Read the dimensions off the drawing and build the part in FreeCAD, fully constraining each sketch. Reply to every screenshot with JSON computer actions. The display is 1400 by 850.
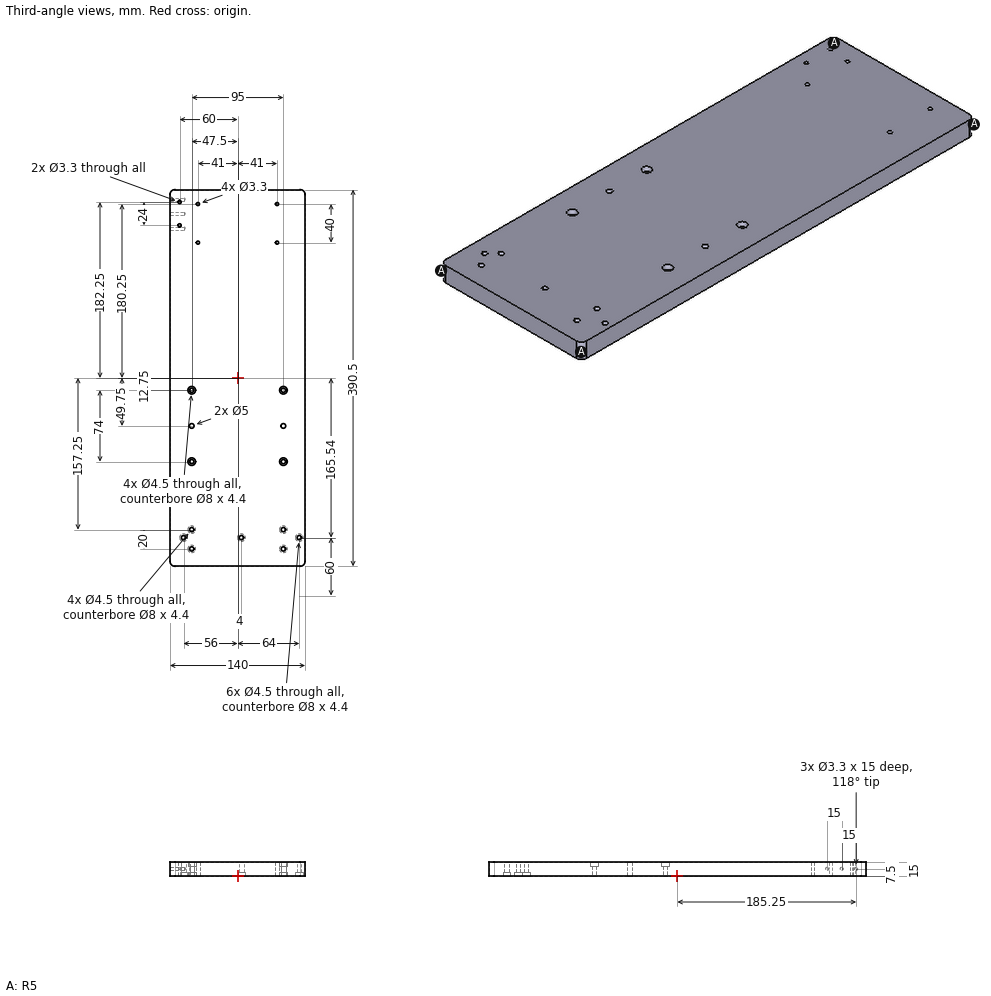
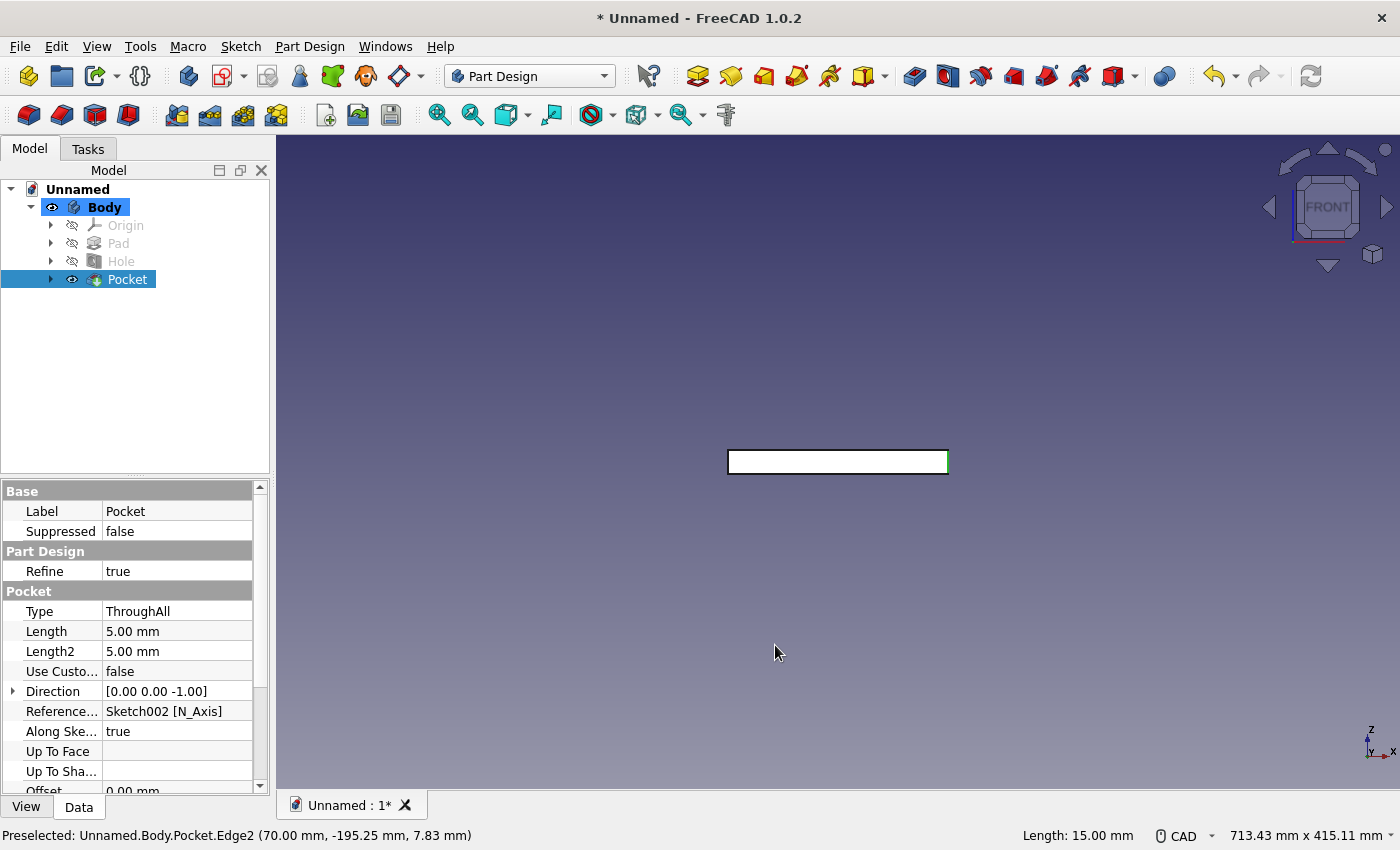
{"action": "key", "text": "v f"}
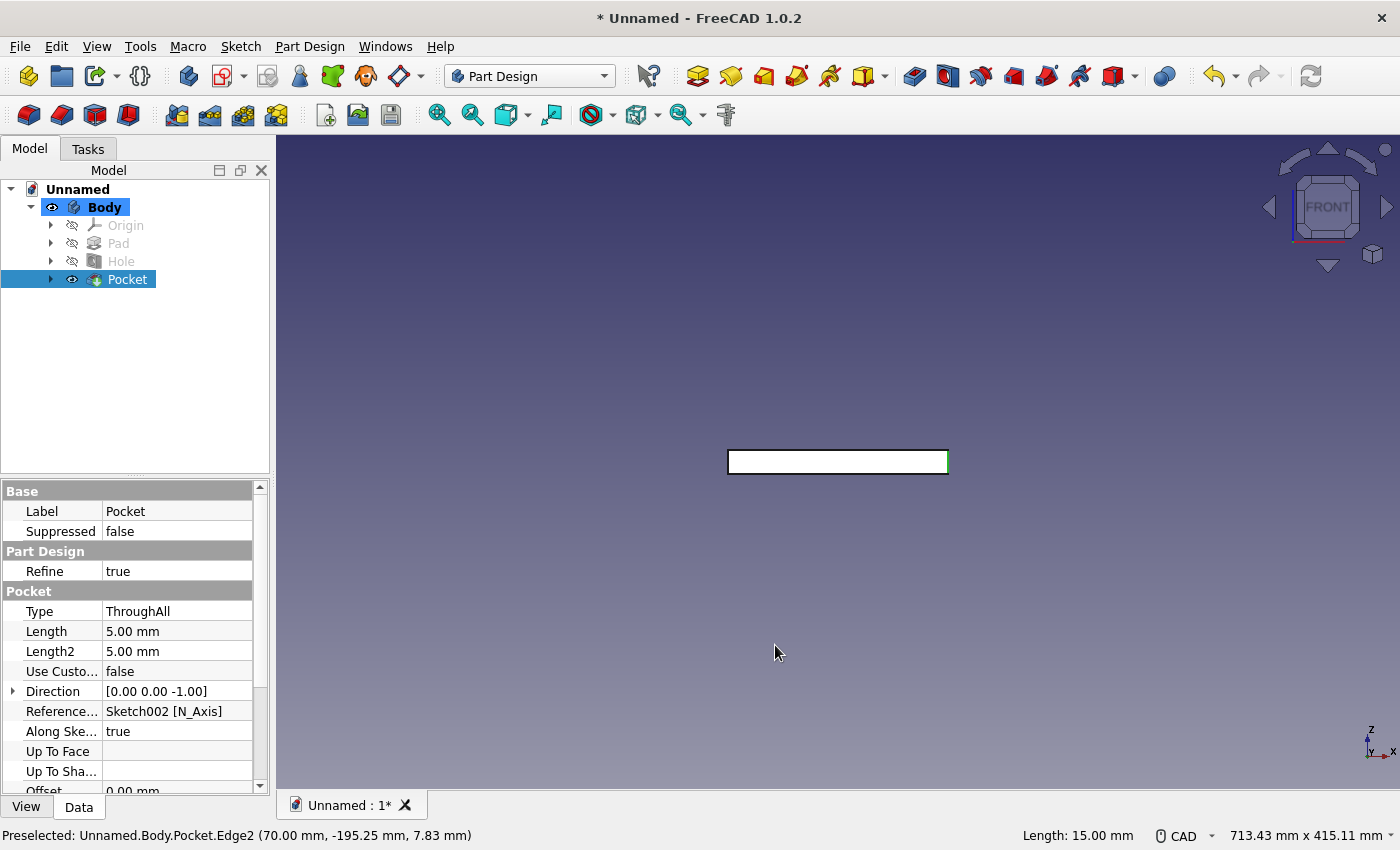
{"action": "left_click", "coordinate": [728, 461], "text": "ctrl"}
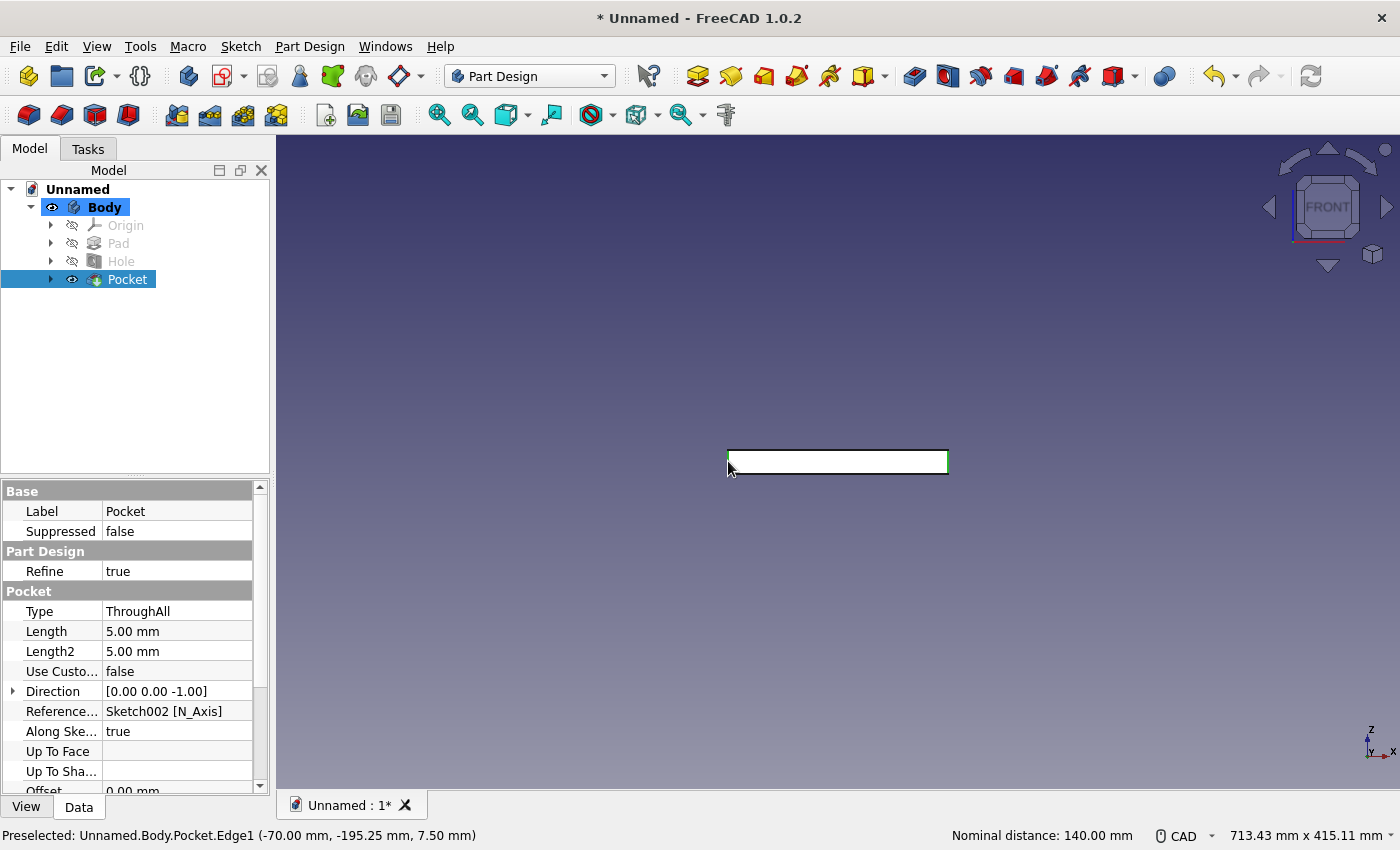
{"action": "key", "text": "3"}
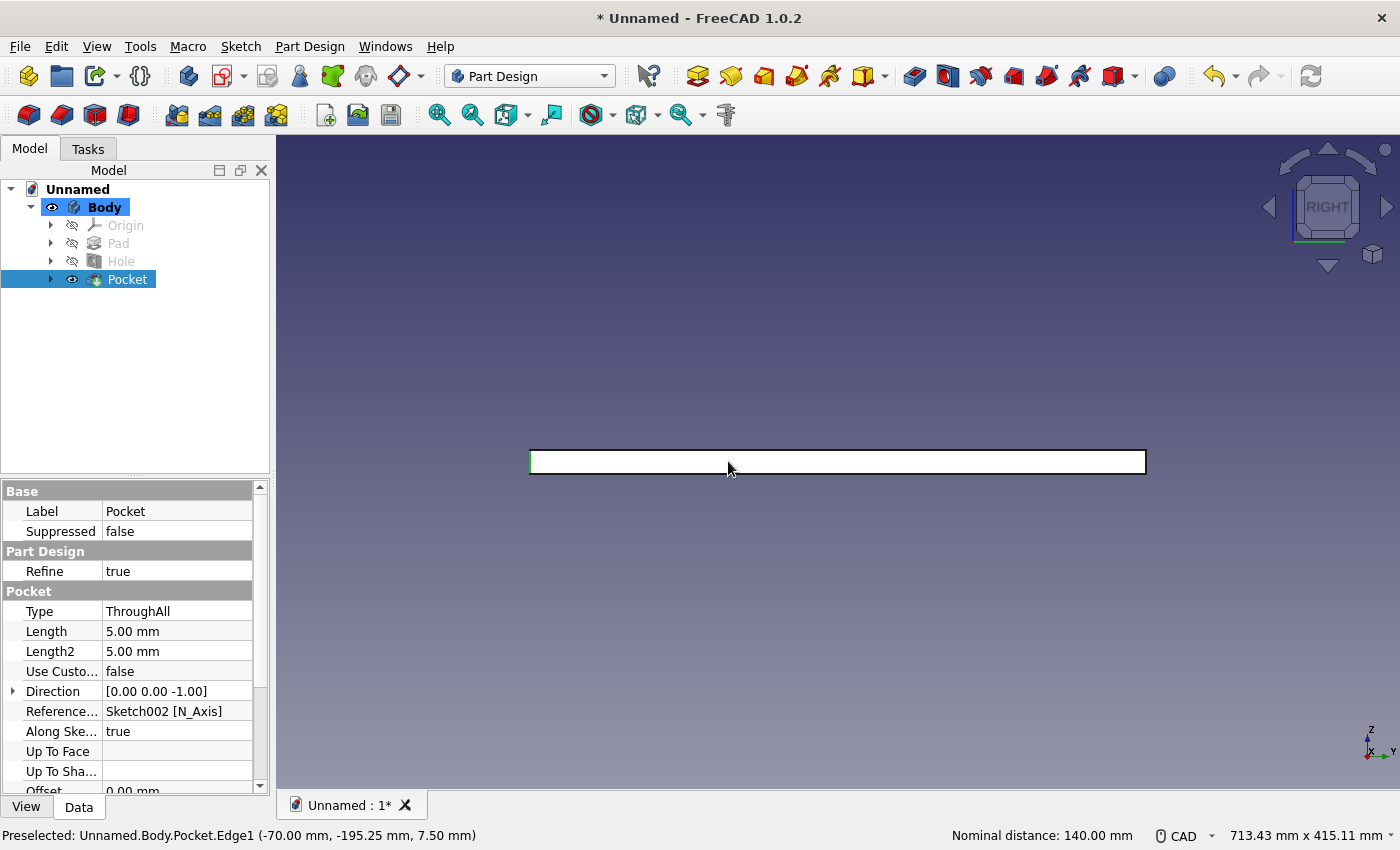
{"action": "left_click", "coordinate": [1146, 461], "text": "ctrl"}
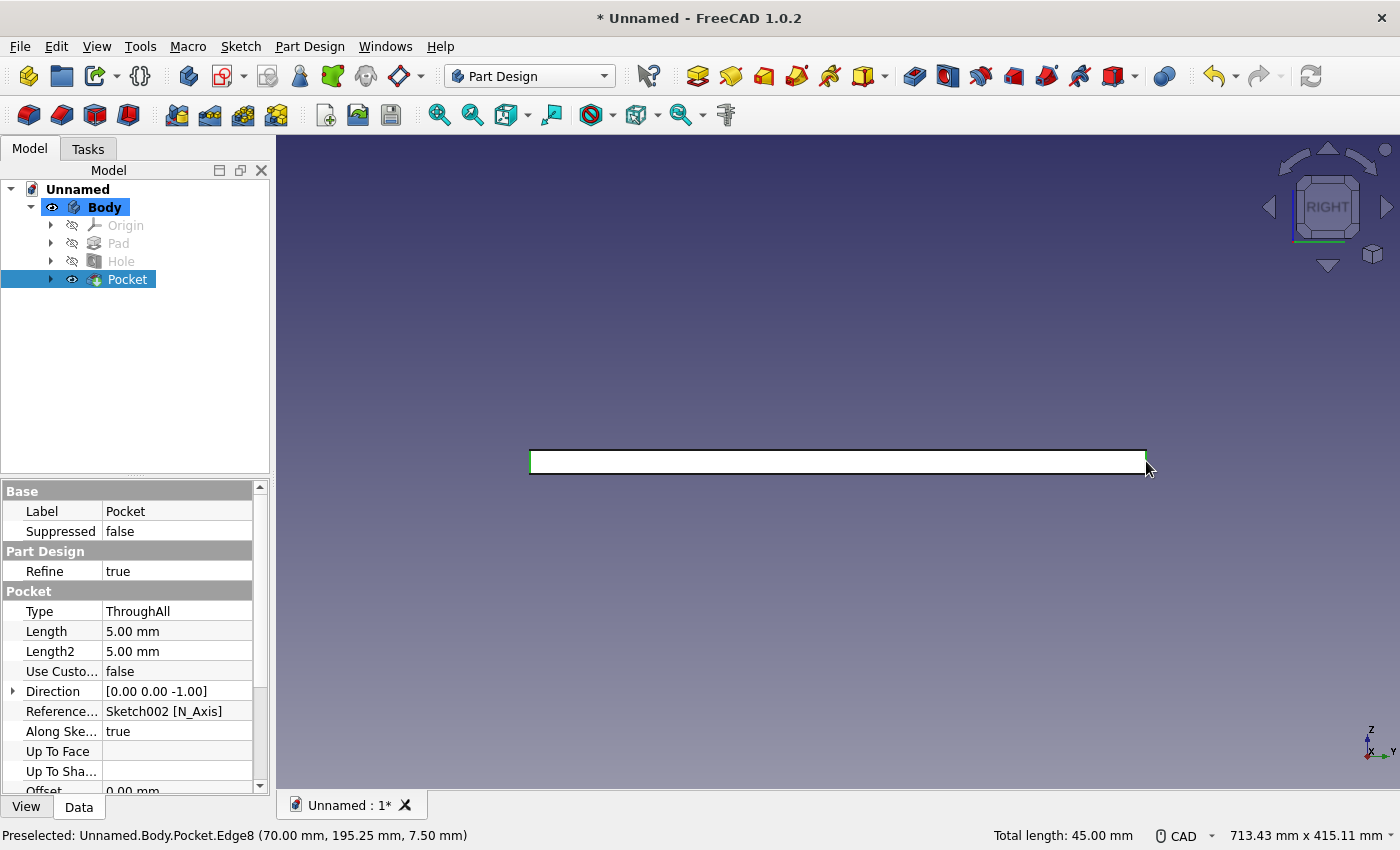
{"action": "key", "text": "5"}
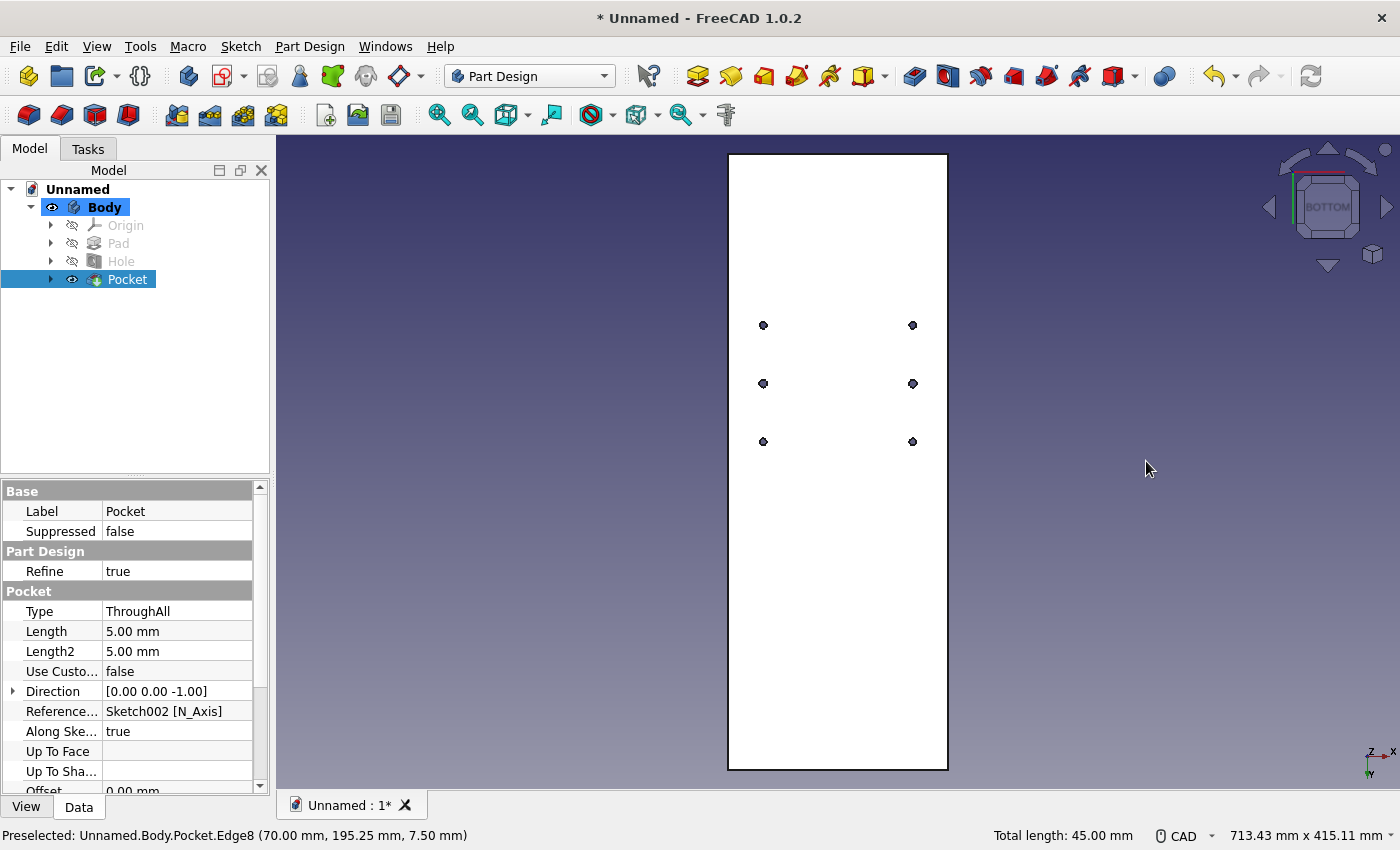
{"action": "key", "text": "4"}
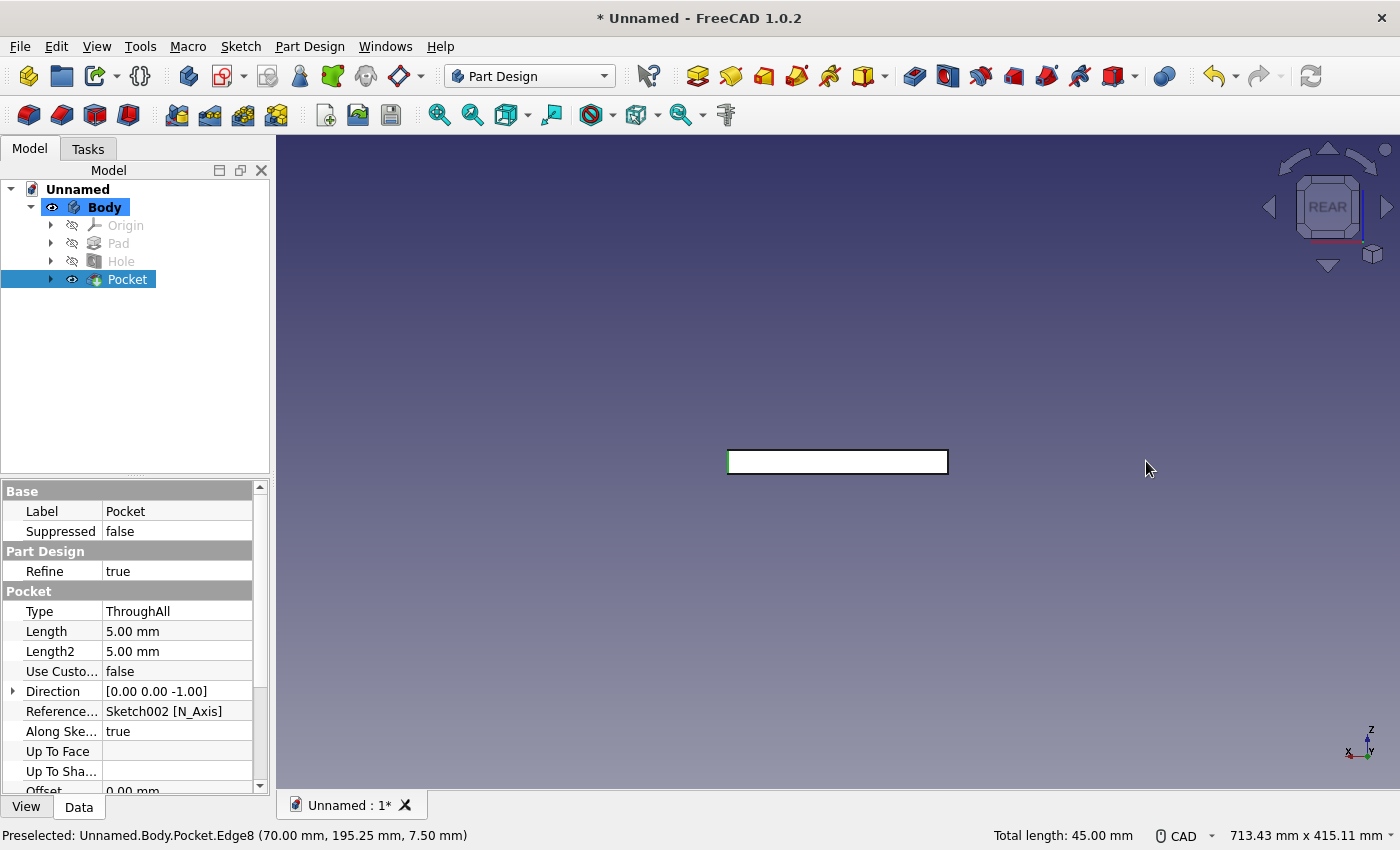
{"action": "left_click", "coordinate": [440, 116]}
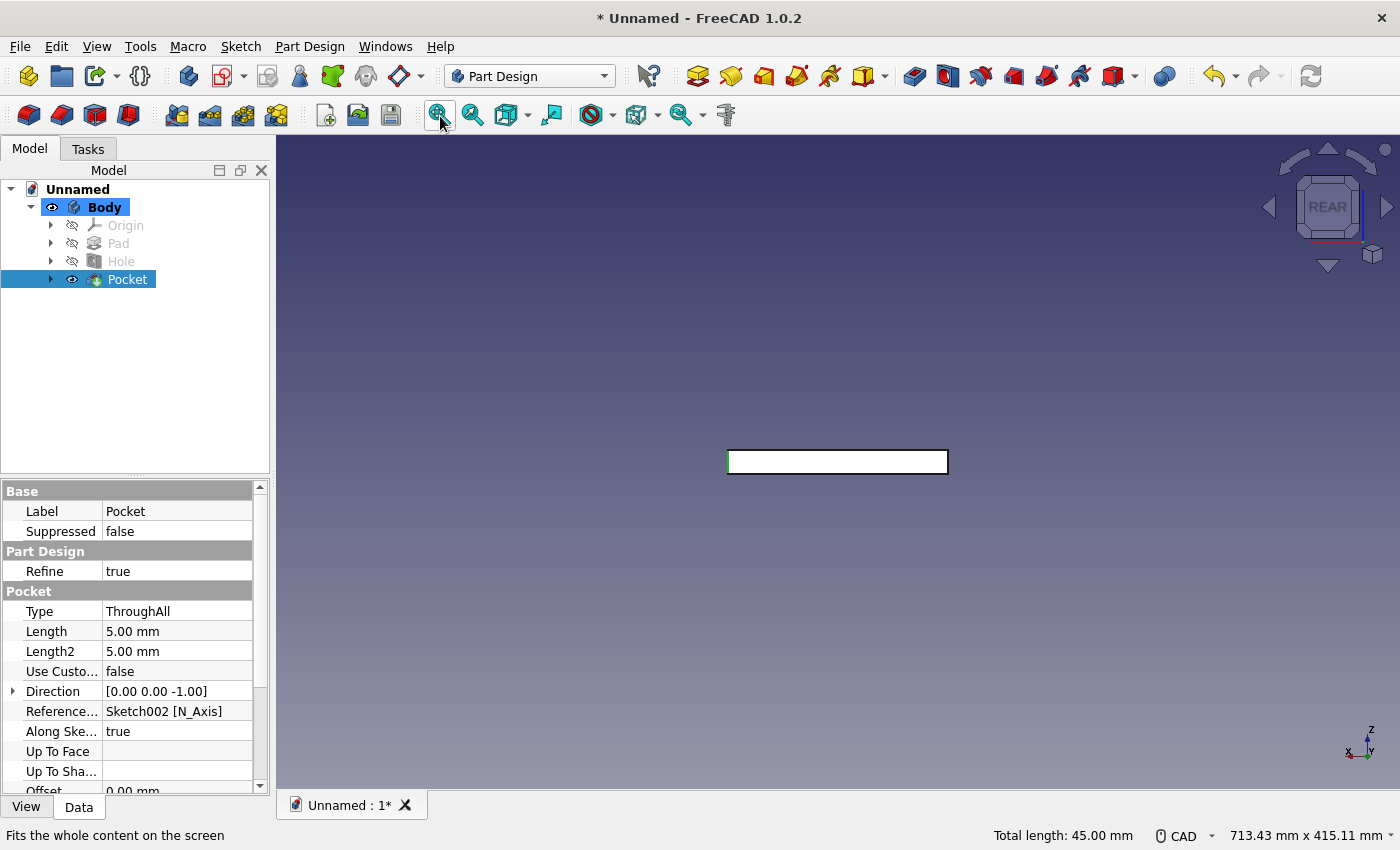
{"action": "left_click", "coordinate": [948, 461], "text": "ctrl"}